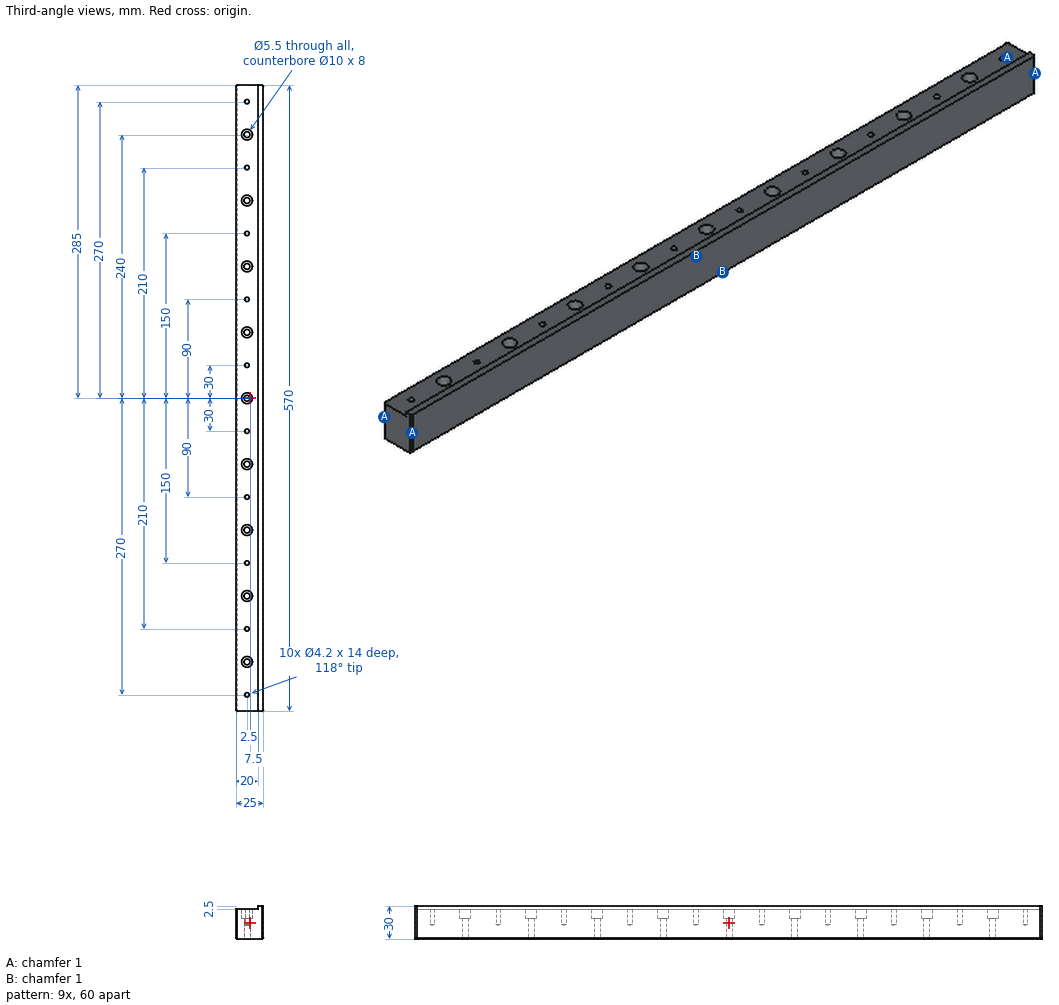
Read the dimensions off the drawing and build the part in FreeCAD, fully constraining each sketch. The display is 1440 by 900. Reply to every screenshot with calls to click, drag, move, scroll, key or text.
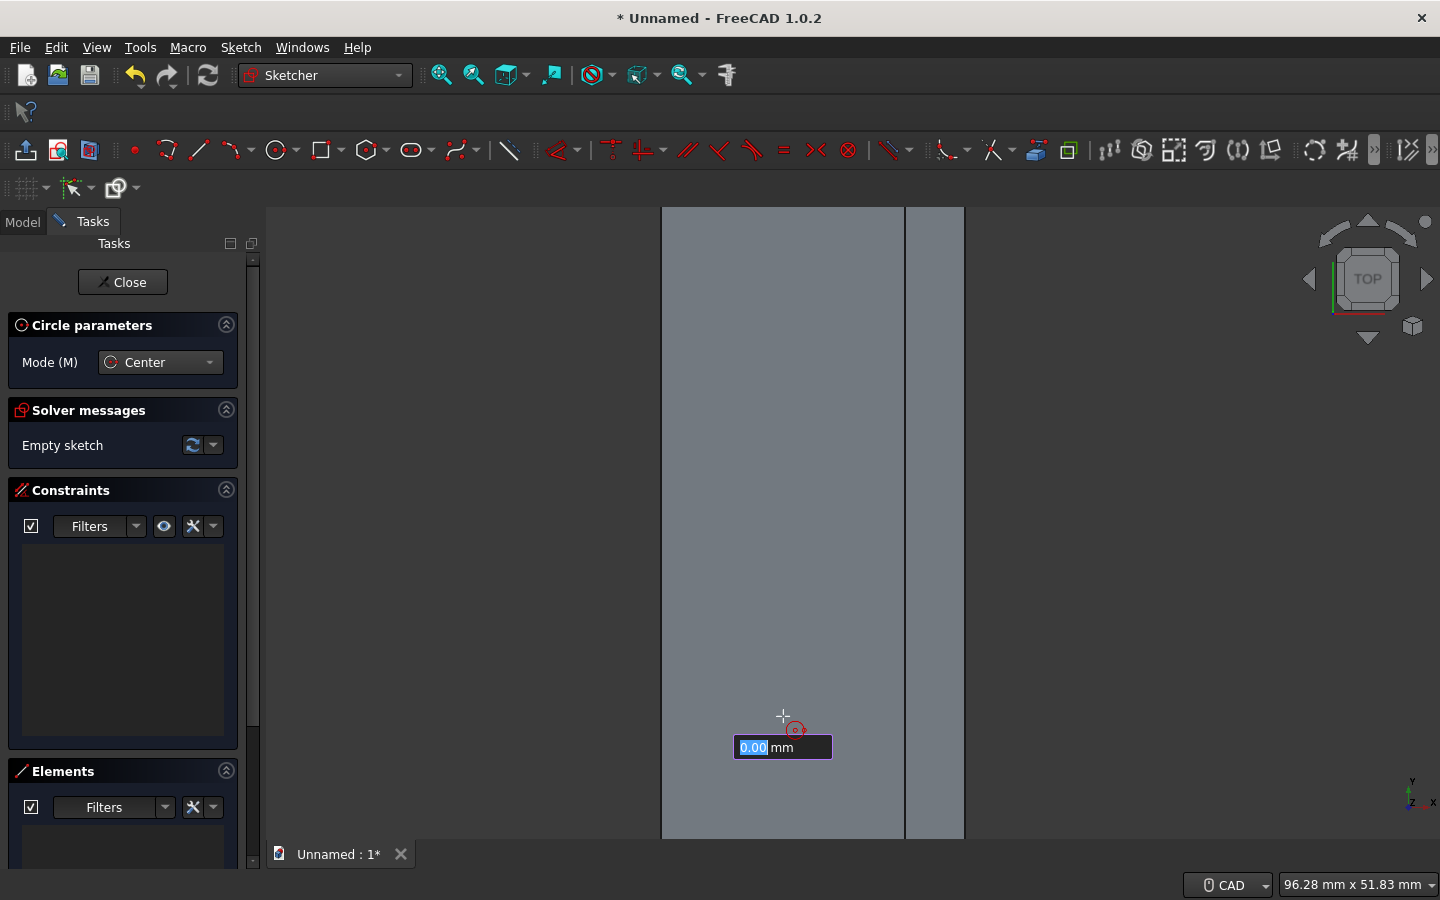
scroll(784, 724, down, 14)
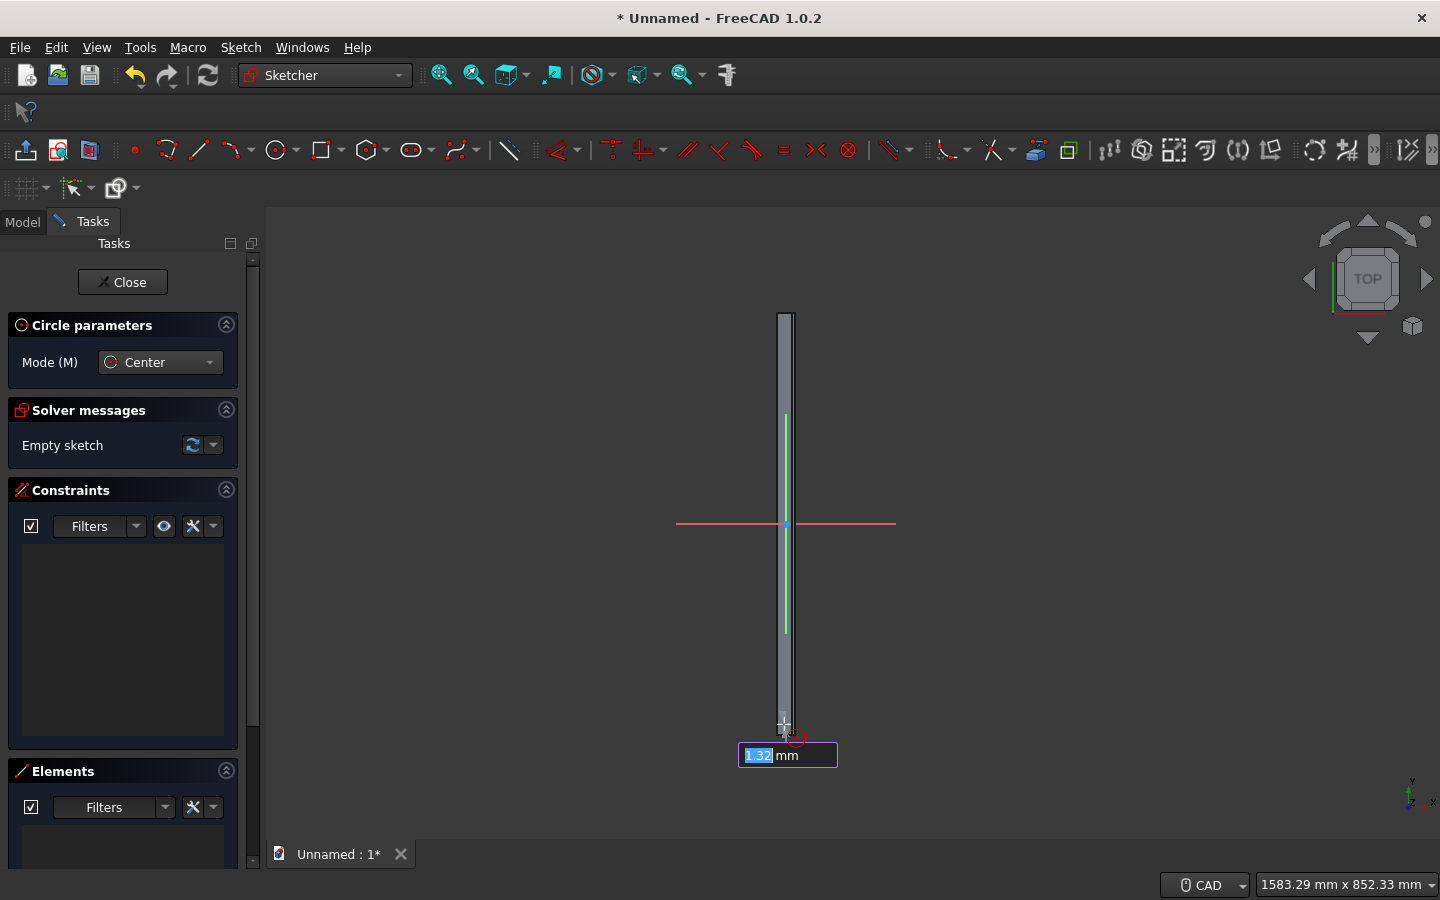
scroll(783, 723, up, 9)
move(782, 720)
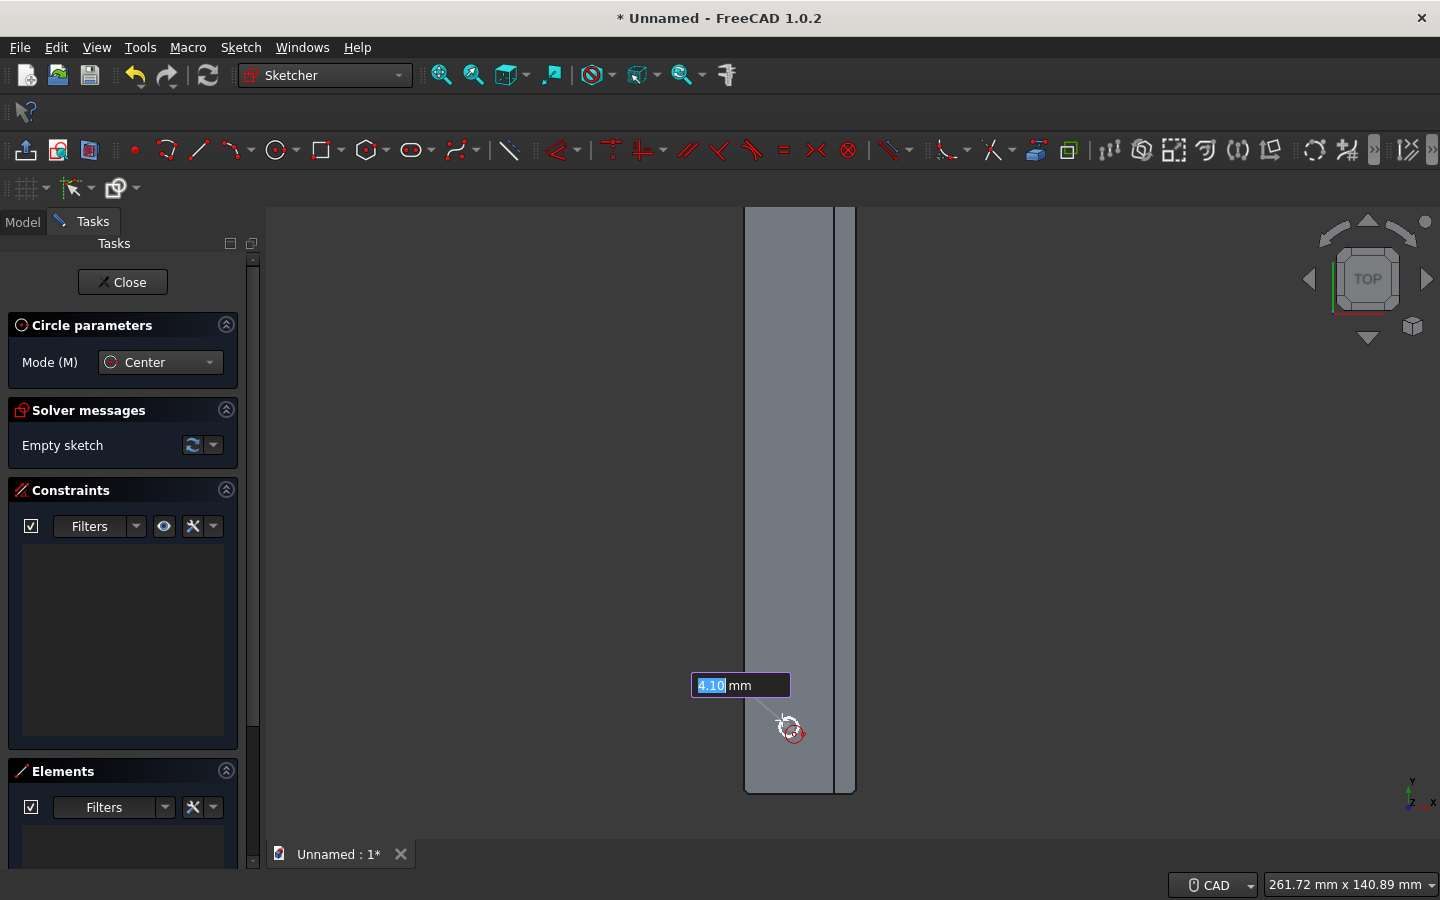
text(4.2)
key(Return)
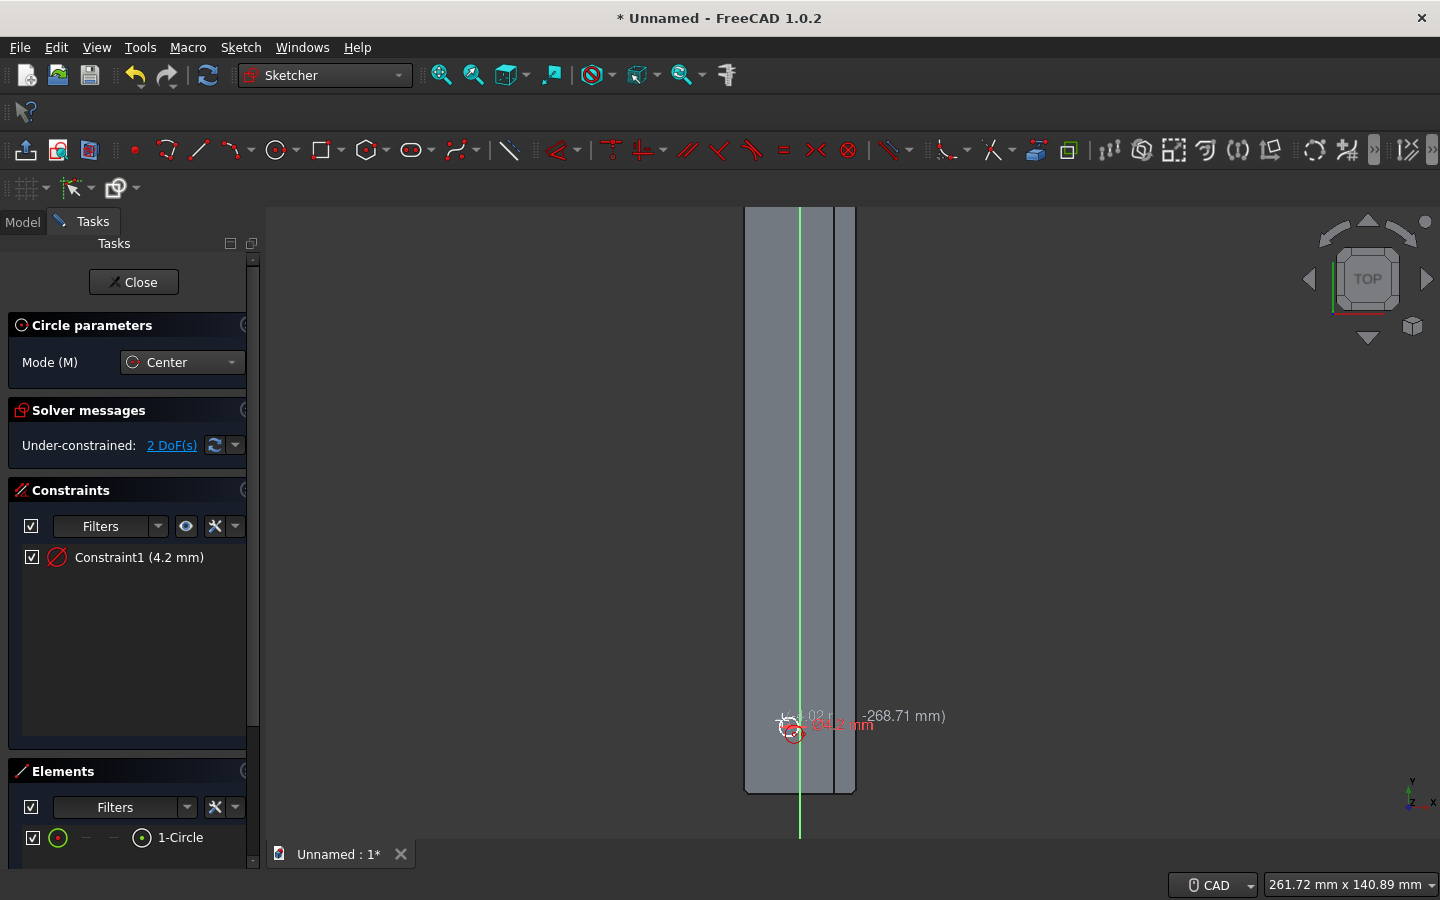
scroll(789, 458, up, 5)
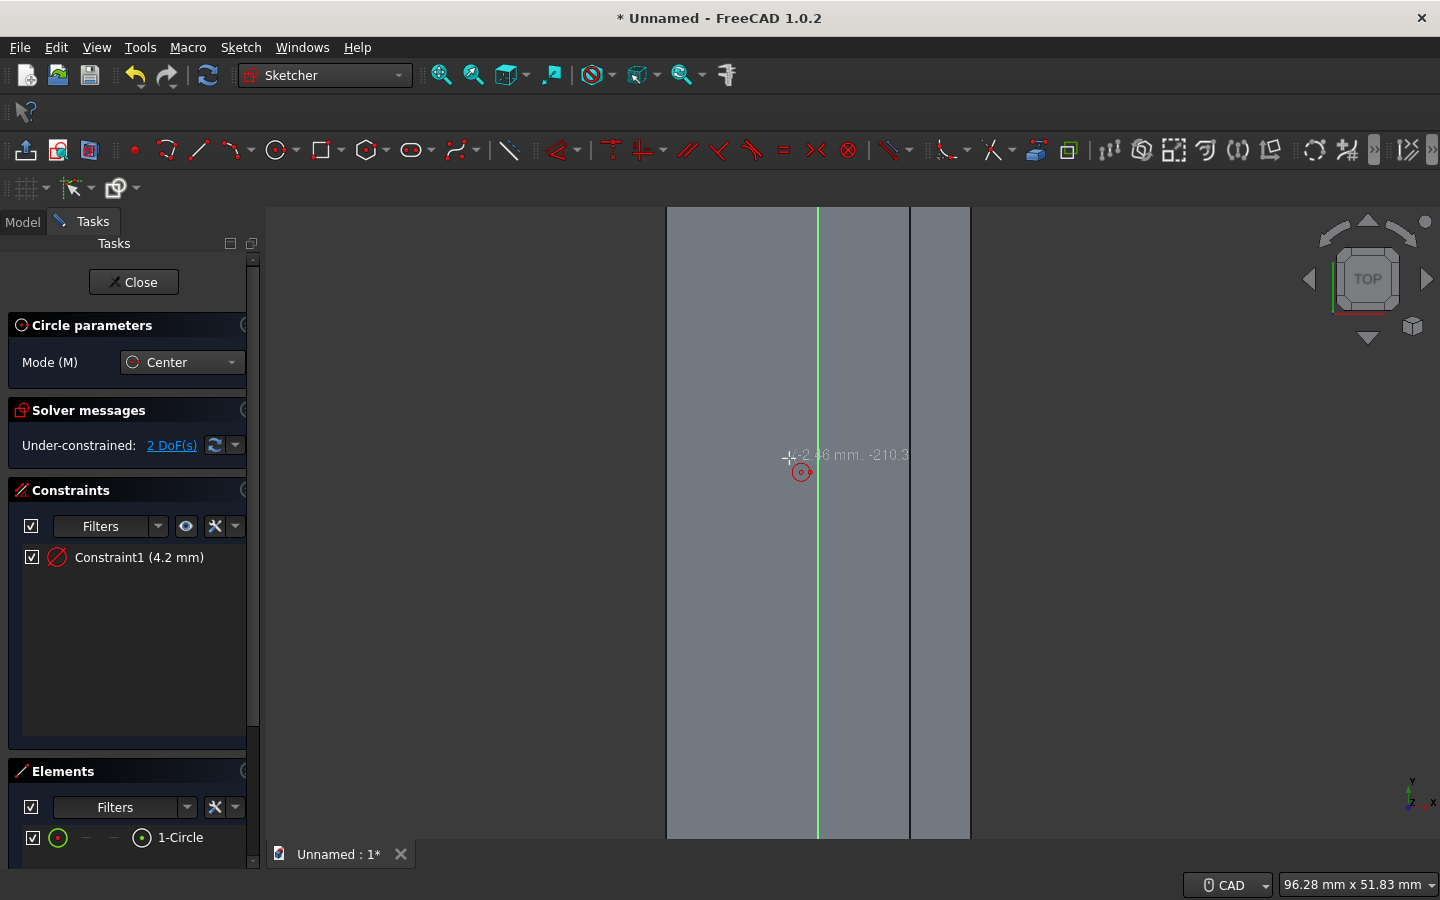
click(788, 456)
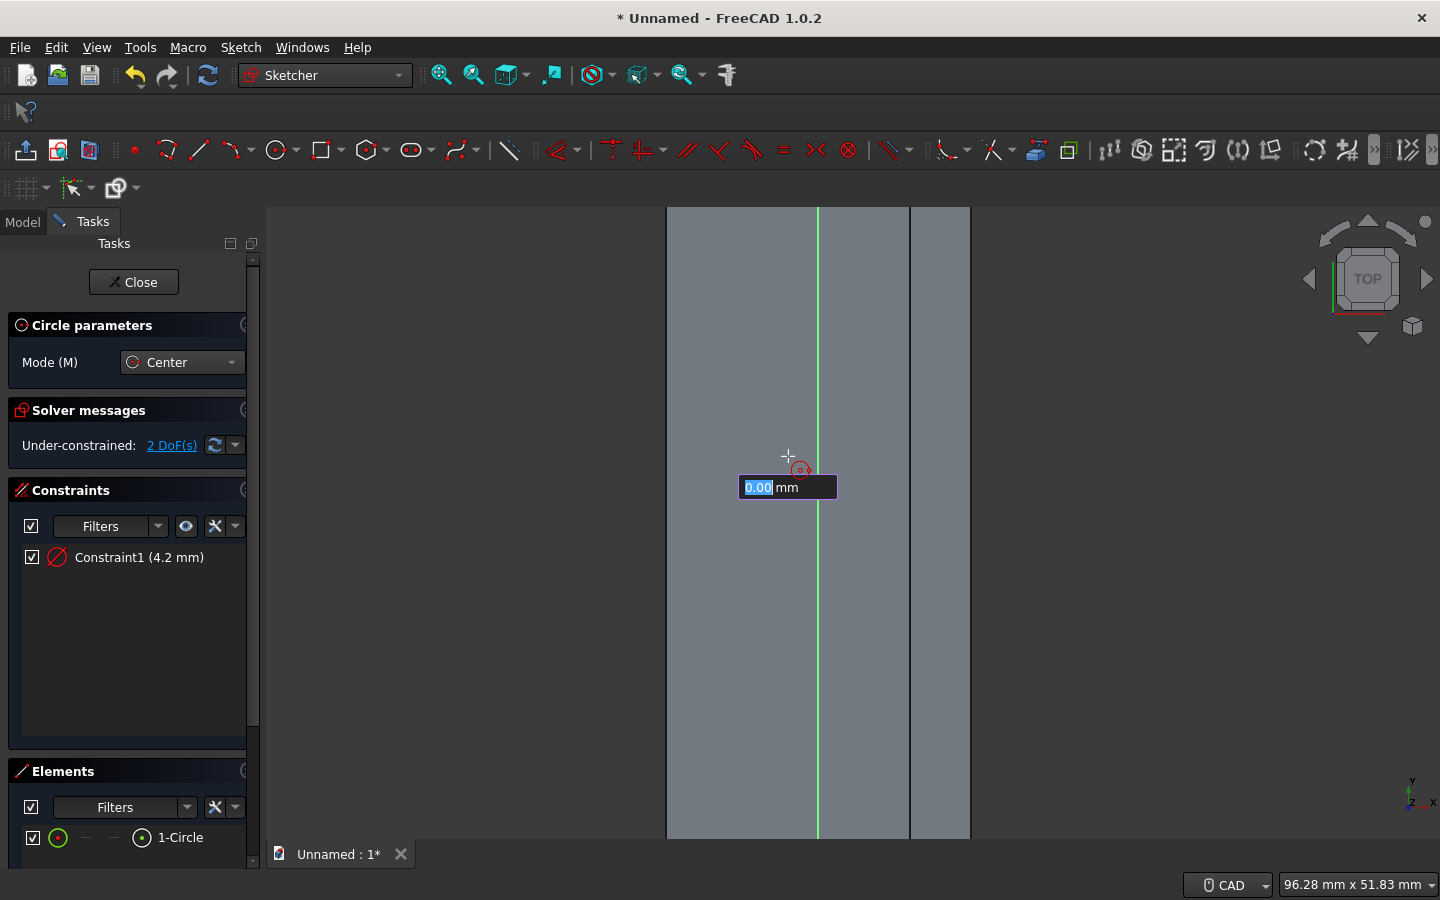
scroll(784, 693, down, 14)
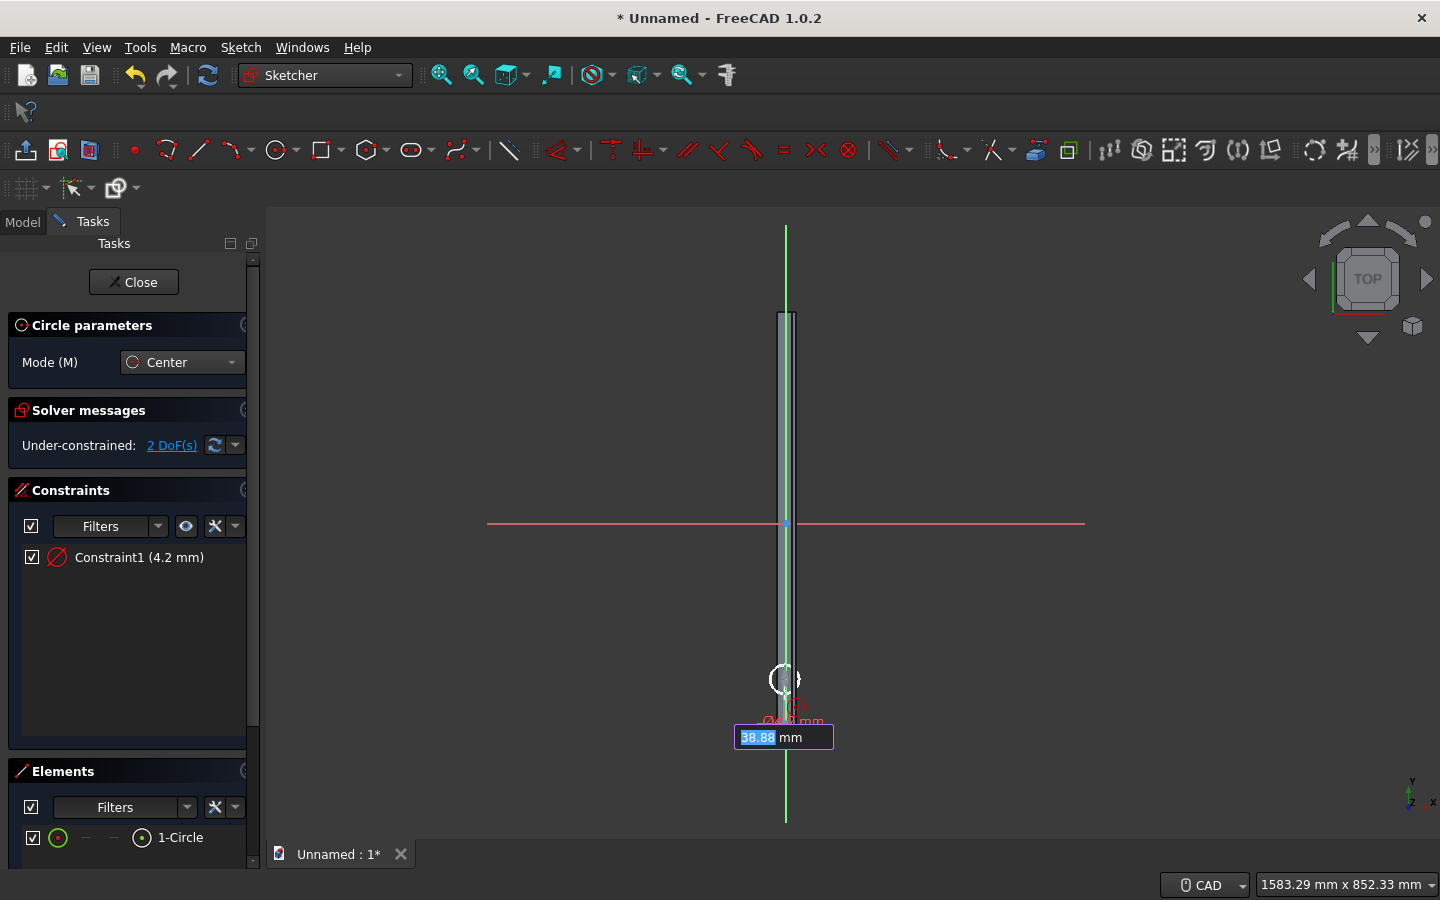
scroll(784, 678, up, 9)
move(779, 676)